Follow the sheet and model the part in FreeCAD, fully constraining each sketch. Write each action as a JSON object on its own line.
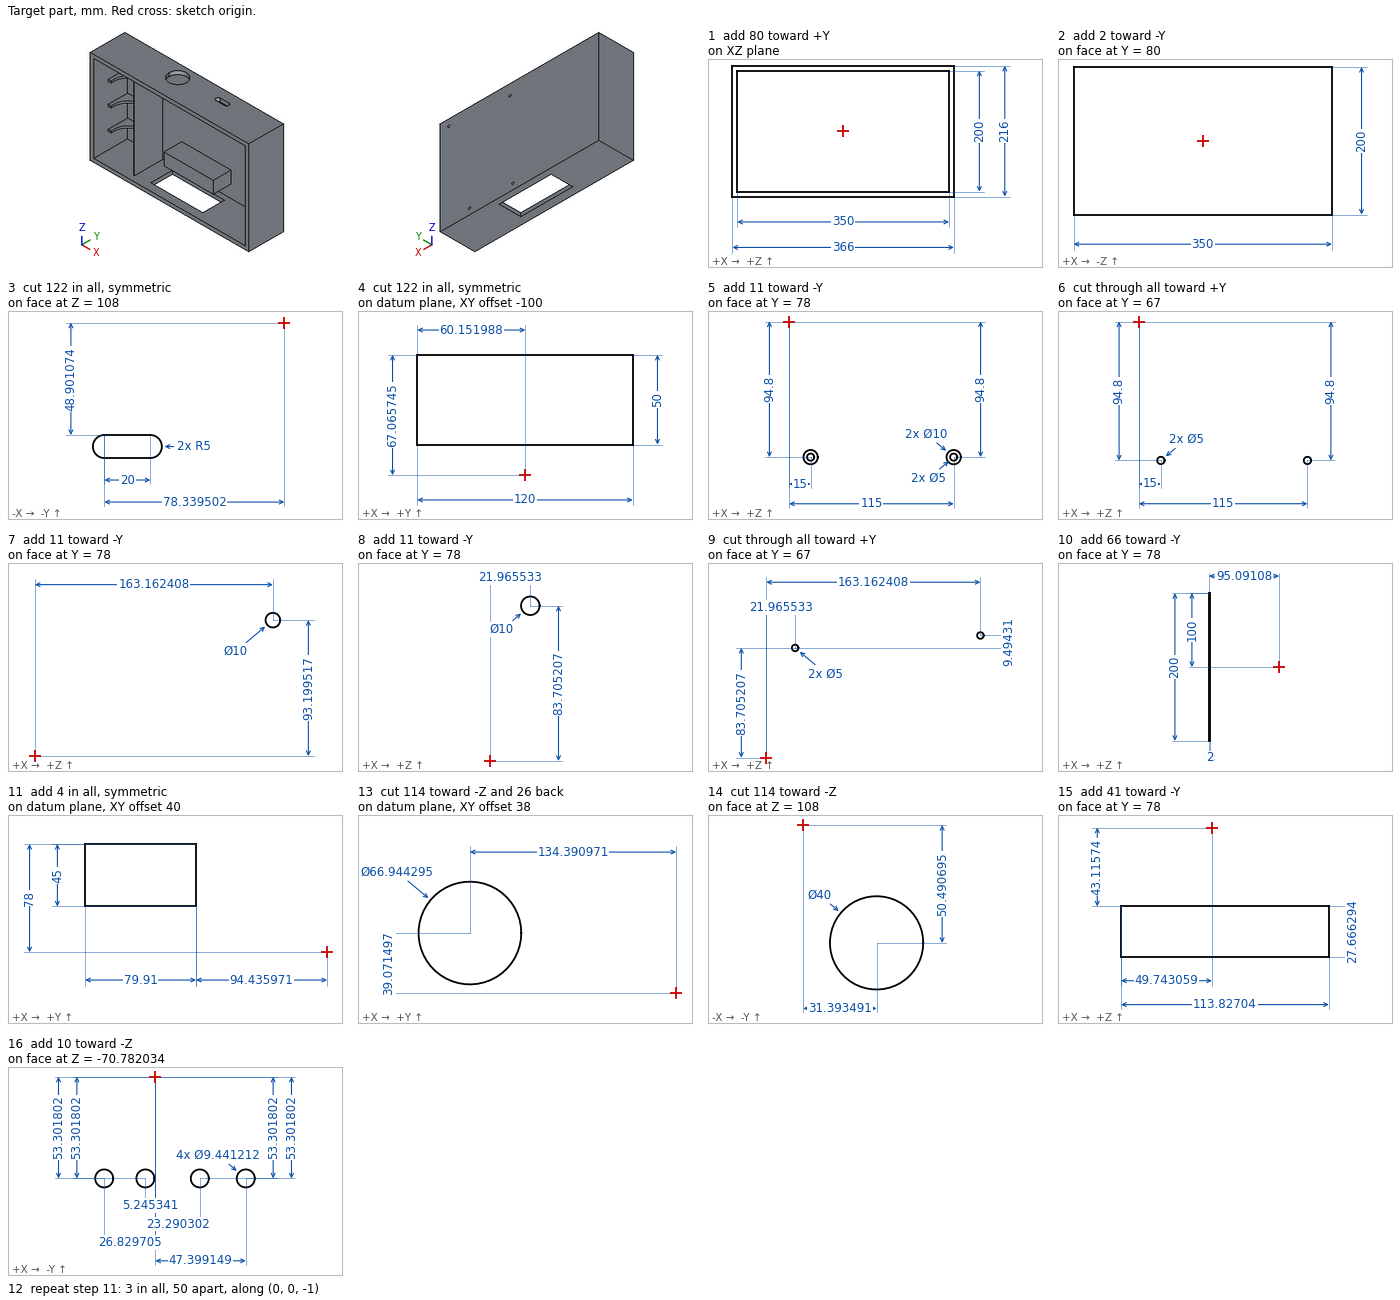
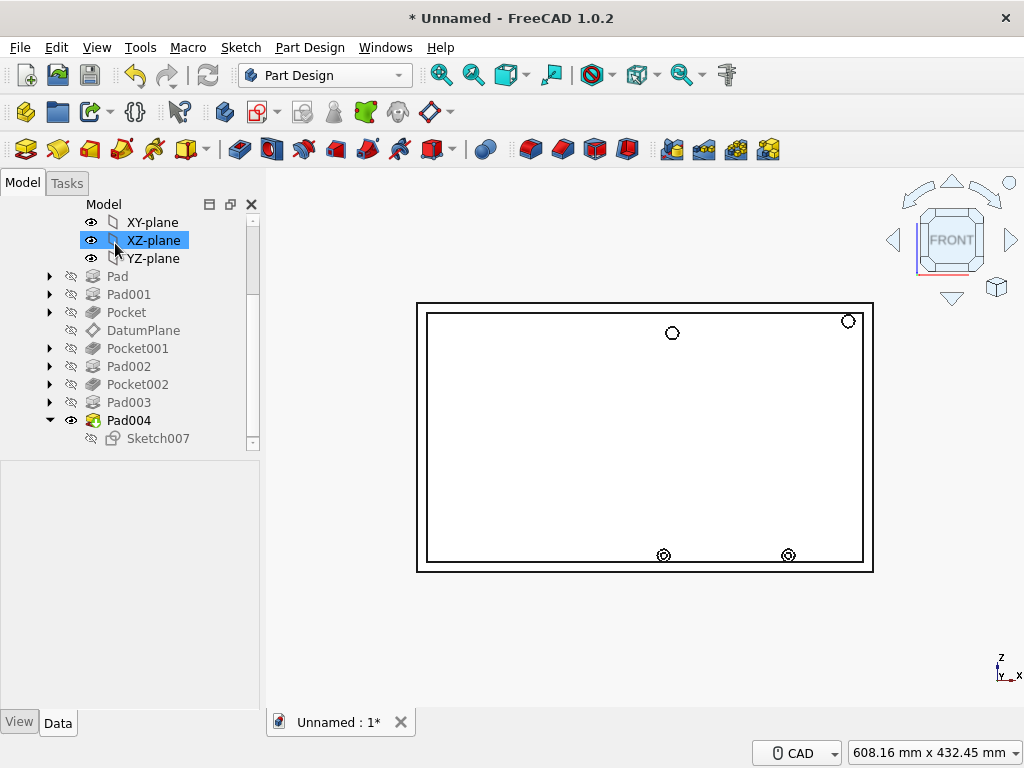
{"action": "scroll", "coordinate": [848, 320], "scroll_direction": "up", "scroll_amount": 4}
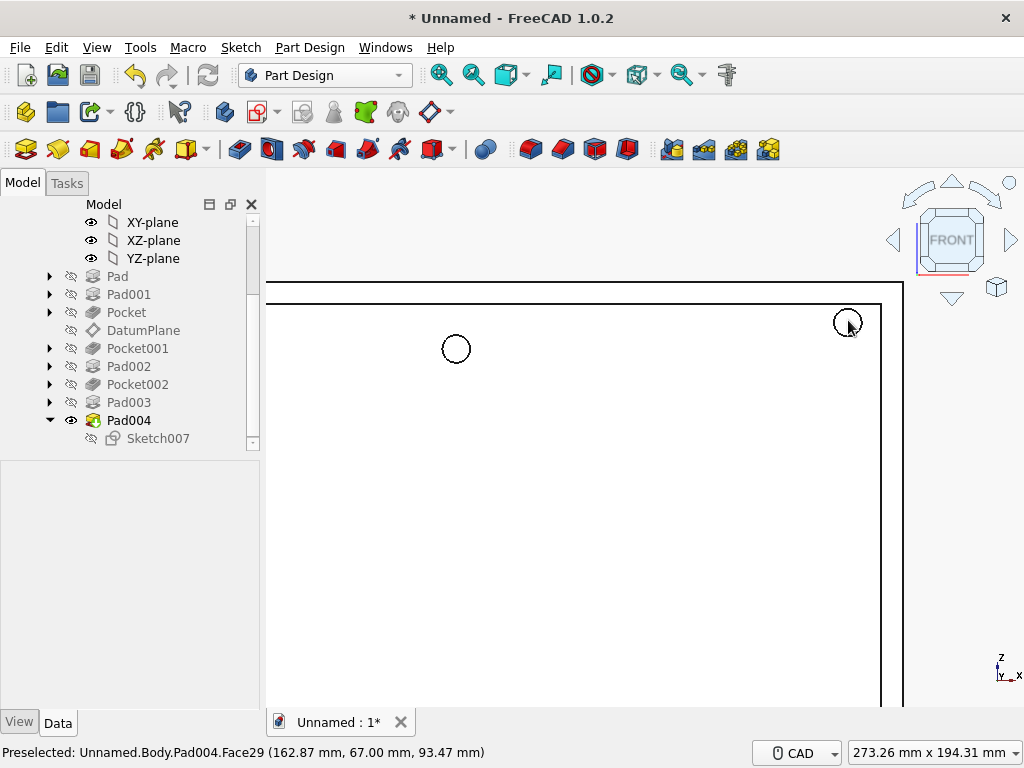
{"action": "left_click", "coordinate": [848, 322]}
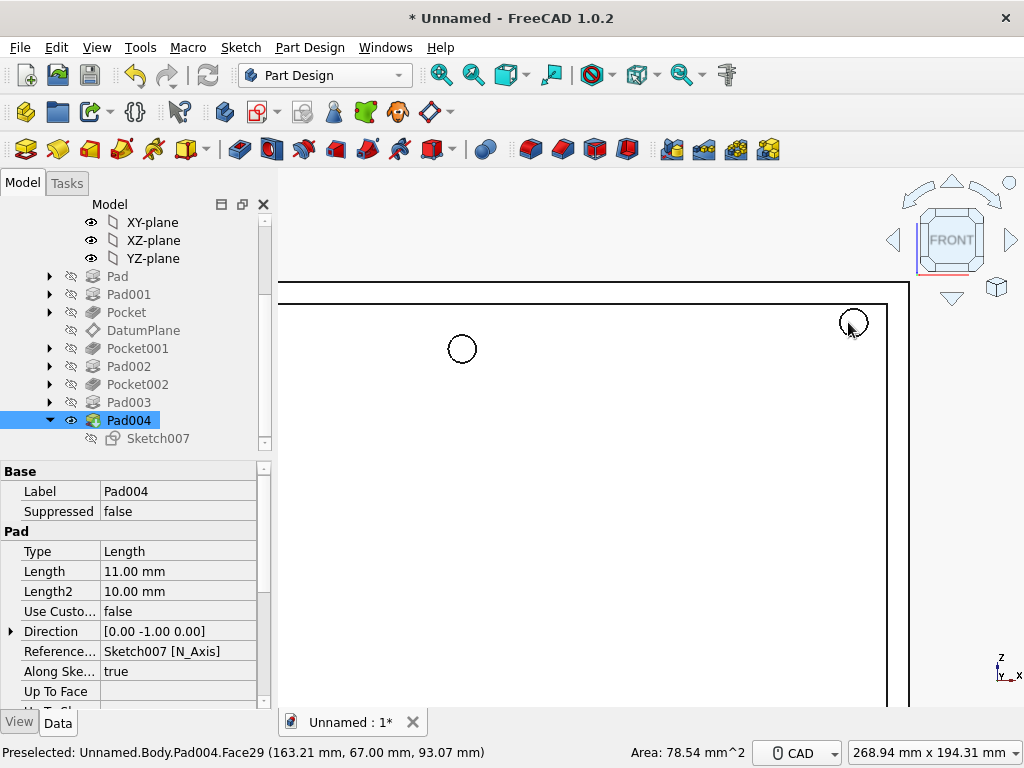
{"action": "left_click", "coordinate": [258, 112]}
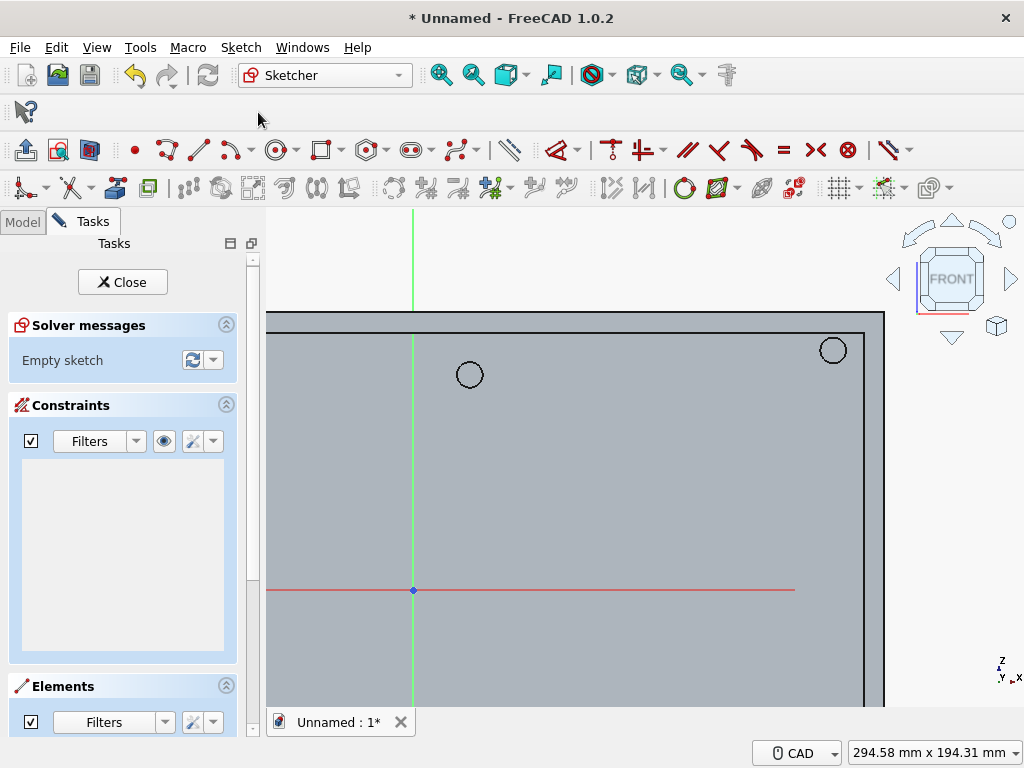
{"action": "scroll", "coordinate": [351, 411], "scroll_direction": "down", "scroll_amount": 1}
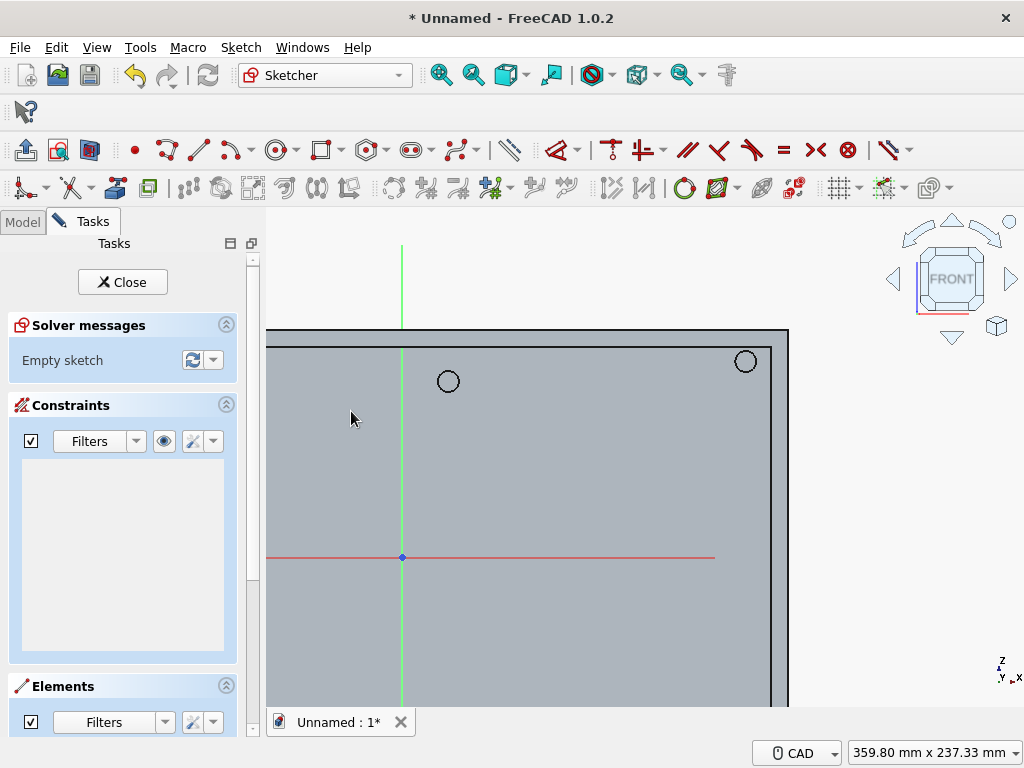
{"action": "key", "text": "g c"}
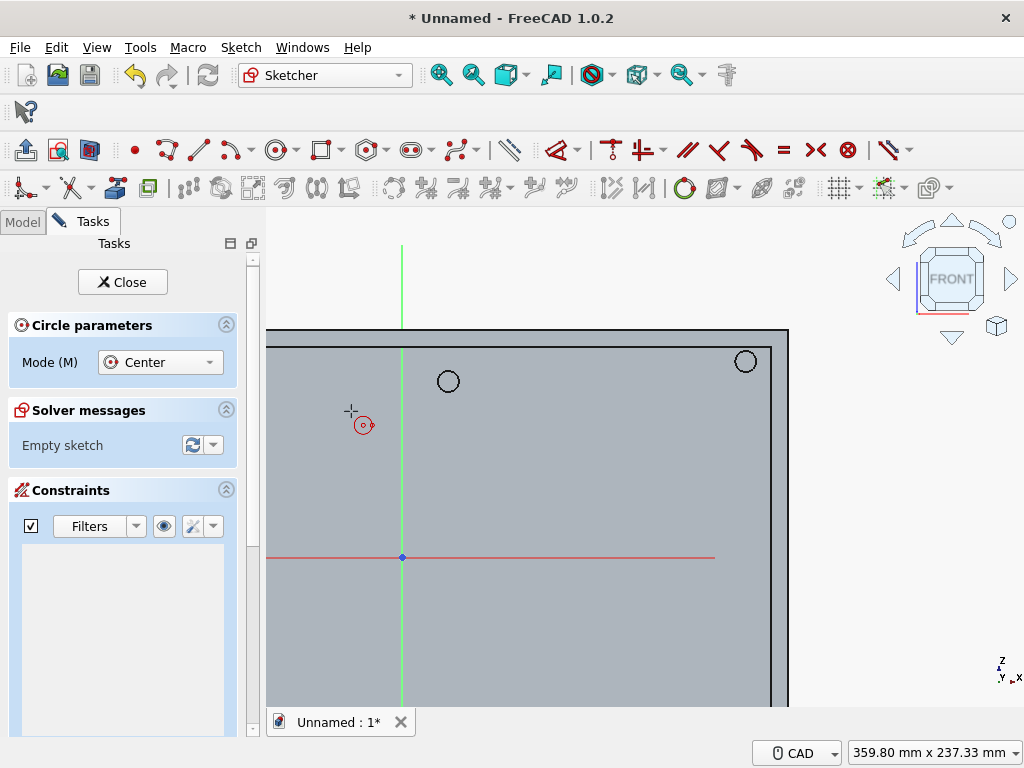
{"action": "scroll", "coordinate": [448, 381], "scroll_direction": "up", "scroll_amount": 8}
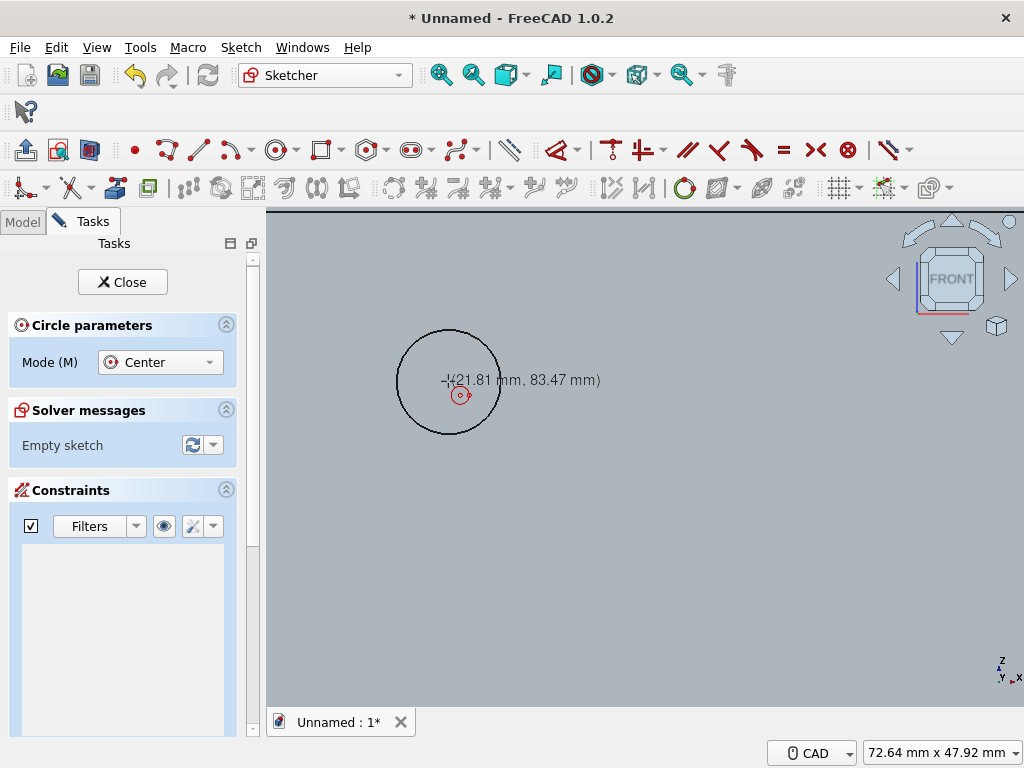
{"action": "scroll", "coordinate": [410, 359], "scroll_direction": "down", "scroll_amount": 7}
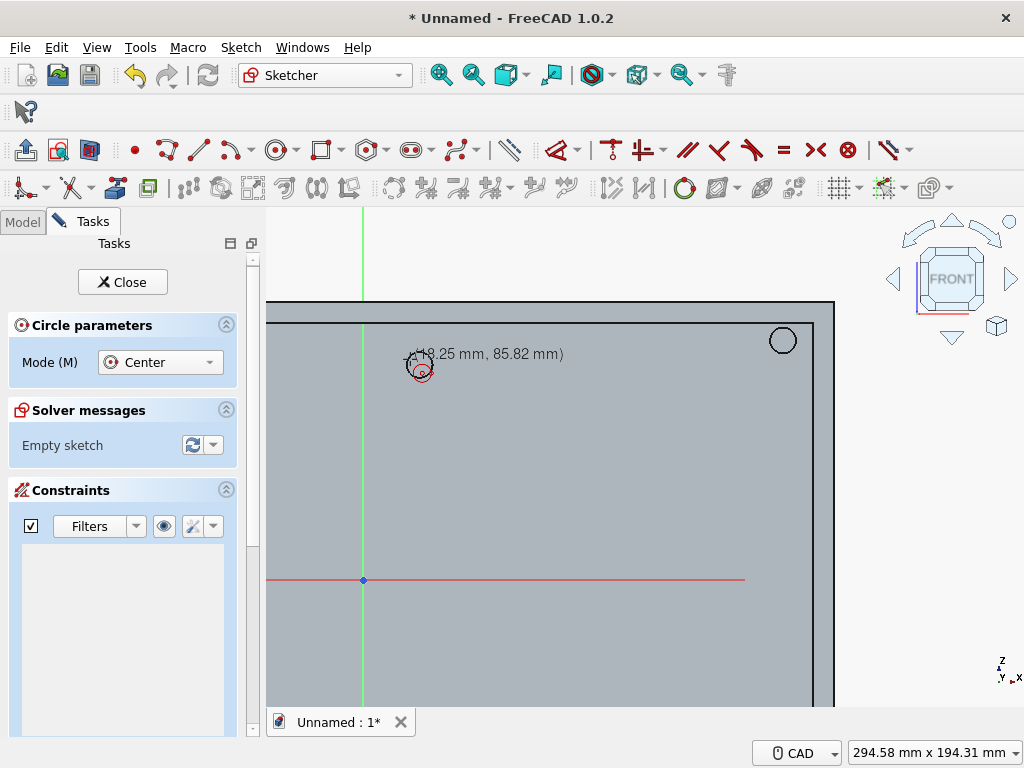
{"action": "left_click", "coordinate": [420, 365]}
{"action": "mouse_move", "coordinate": [424, 360]}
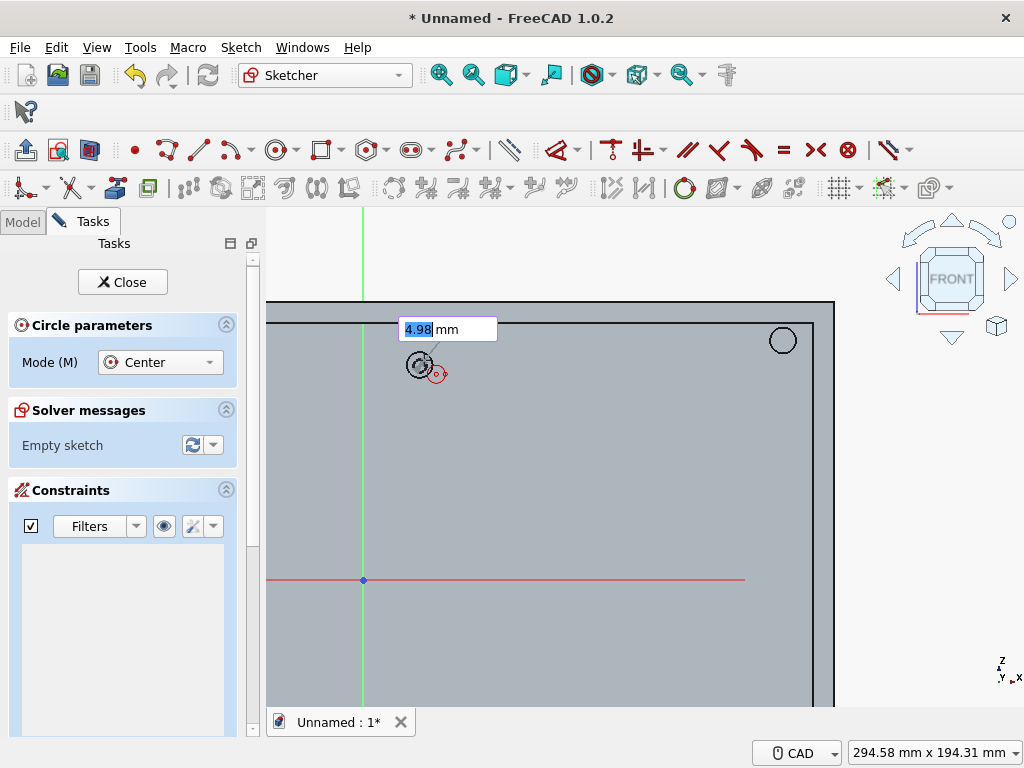
{"action": "type", "text": "5"}
{"action": "key", "text": "Return"}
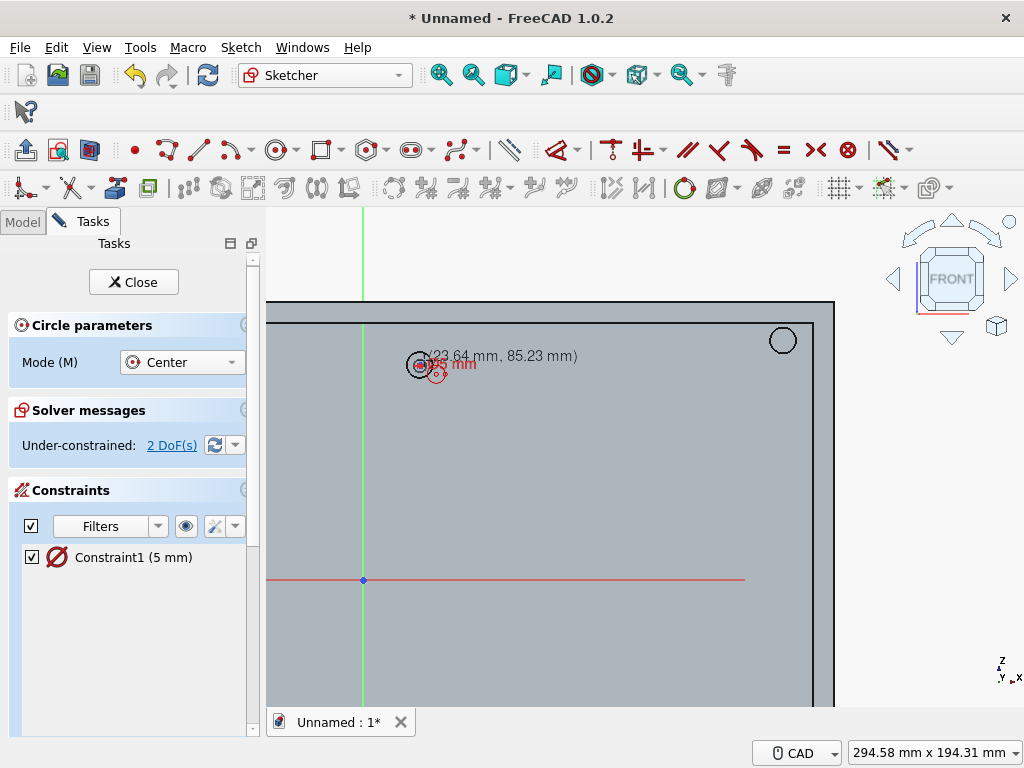
{"action": "scroll", "coordinate": [783, 340], "scroll_direction": "up", "scroll_amount": 7}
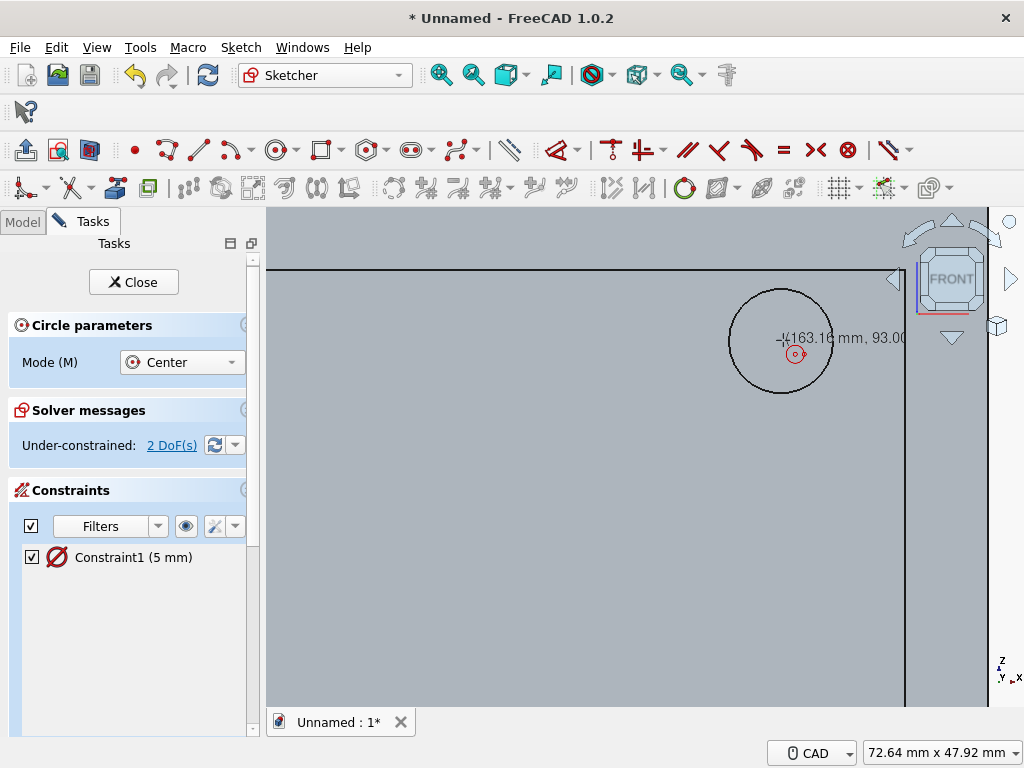
{"action": "scroll", "coordinate": [784, 340], "scroll_direction": "down", "scroll_amount": 7}